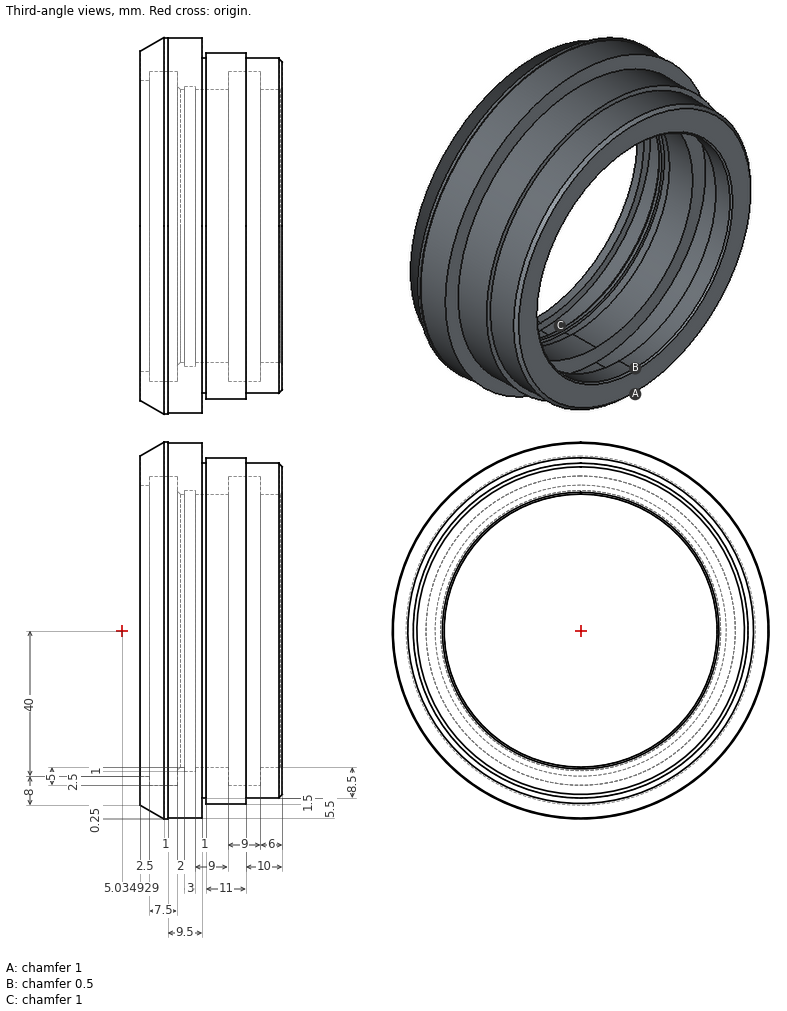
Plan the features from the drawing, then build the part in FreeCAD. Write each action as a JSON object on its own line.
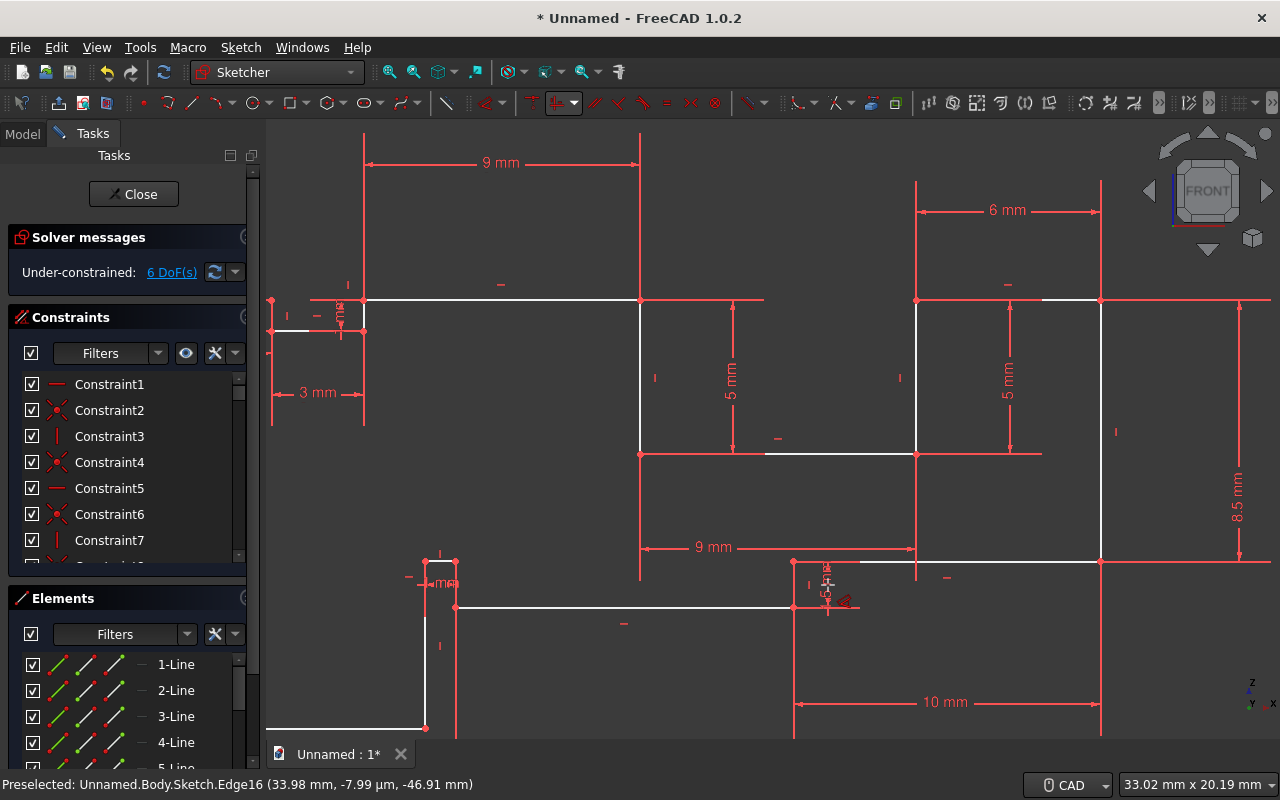
{"action": "left_click", "coordinate": [456, 594]}
{"action": "left_click", "coordinate": [514, 584]}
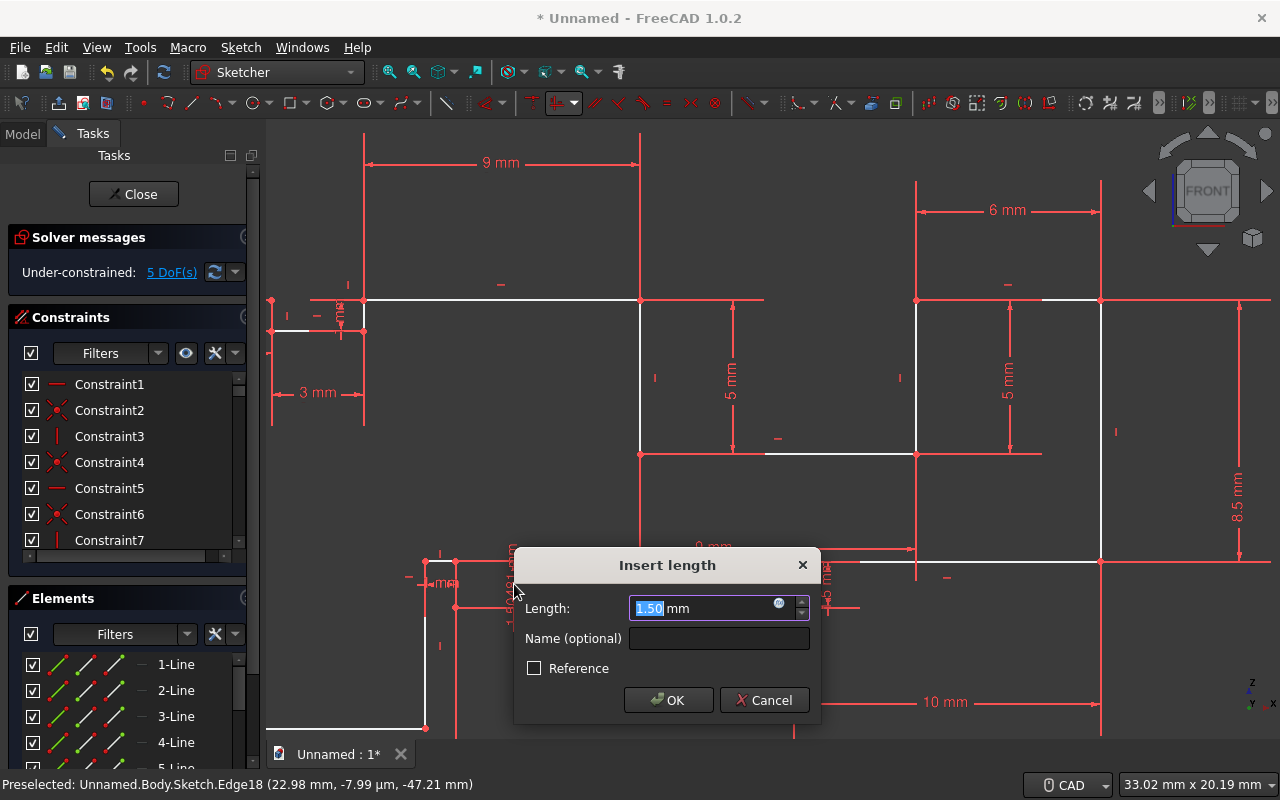
{"action": "type", "text": "1.5"}
{"action": "key", "text": "Return"}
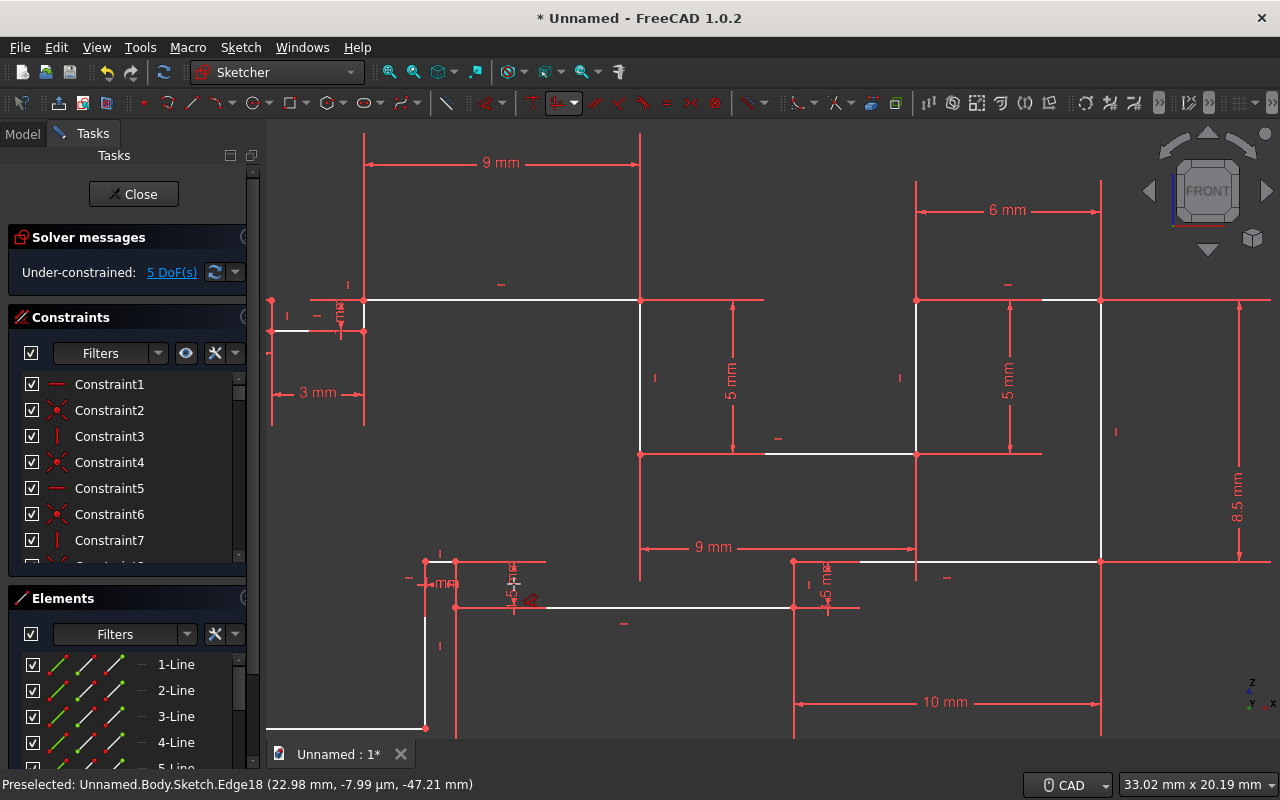
{"action": "left_click", "coordinate": [425, 612]}
{"action": "left_click", "coordinate": [391, 636]}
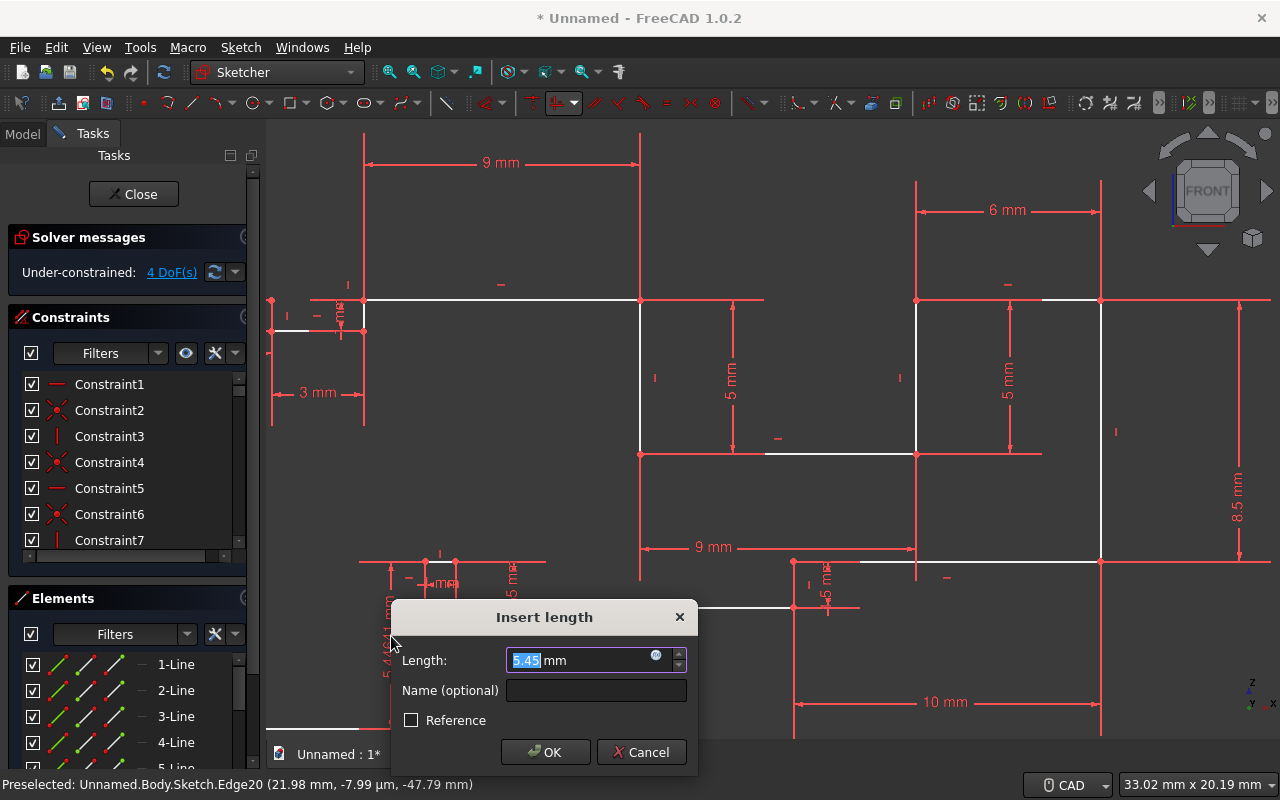
{"action": "type", "text": "5.5"}
{"action": "key", "text": "Return"}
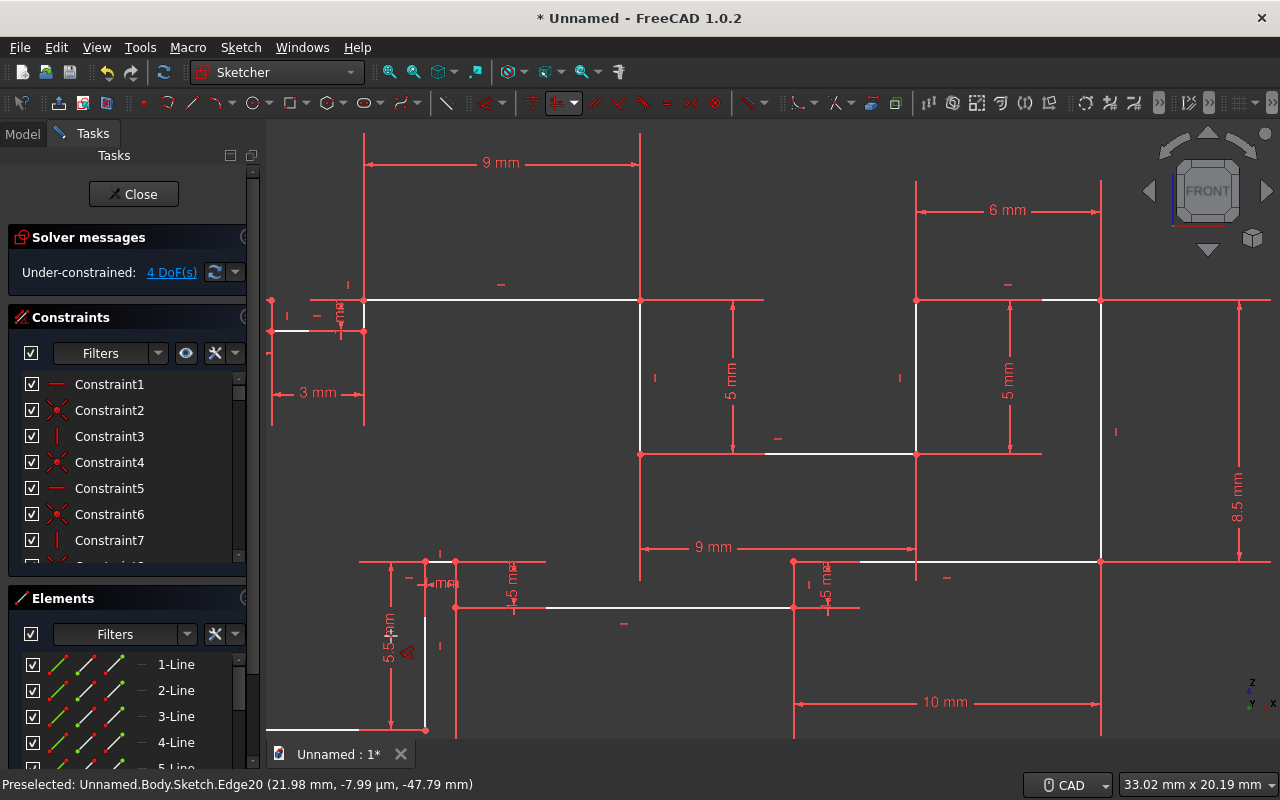
{"action": "scroll", "coordinate": [796, 589], "scroll_direction": "down", "scroll_amount": 7}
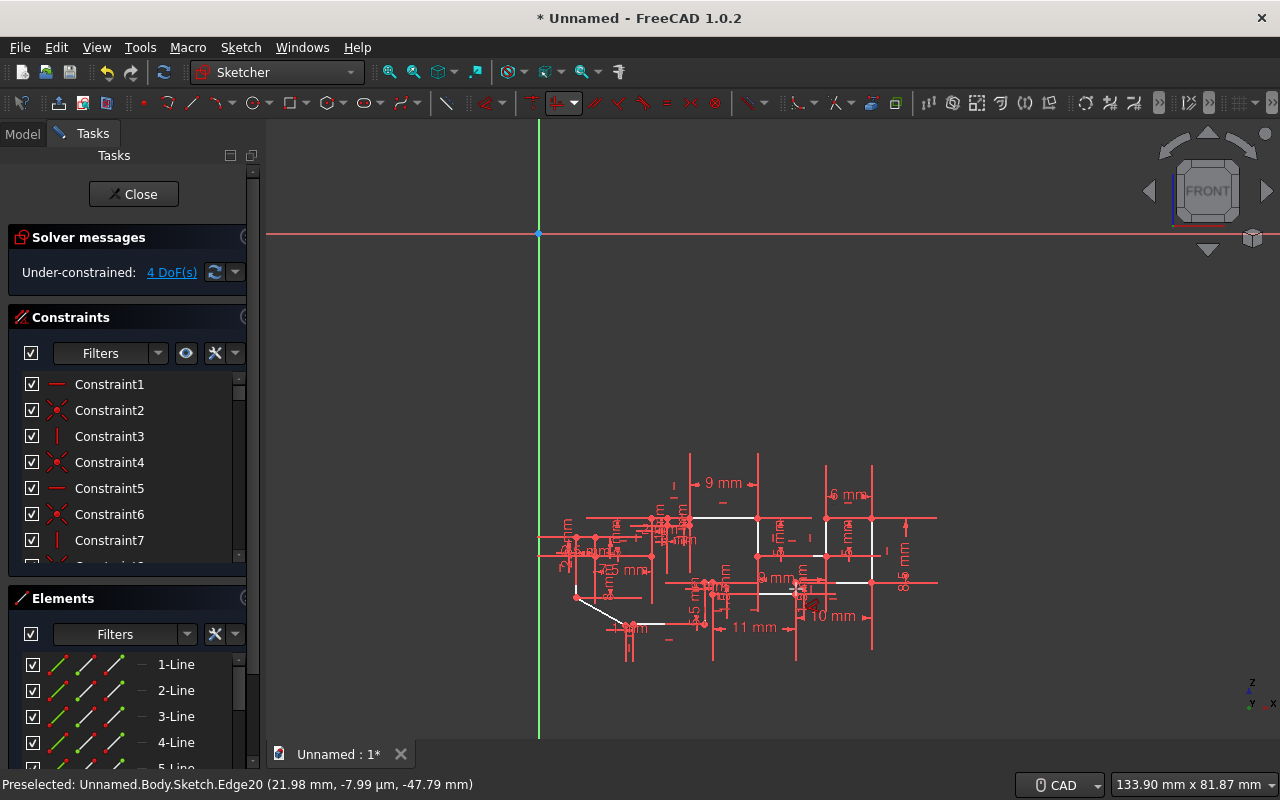
{"action": "left_click", "coordinate": [683, 624]}
{"action": "left_click", "coordinate": [669, 658]}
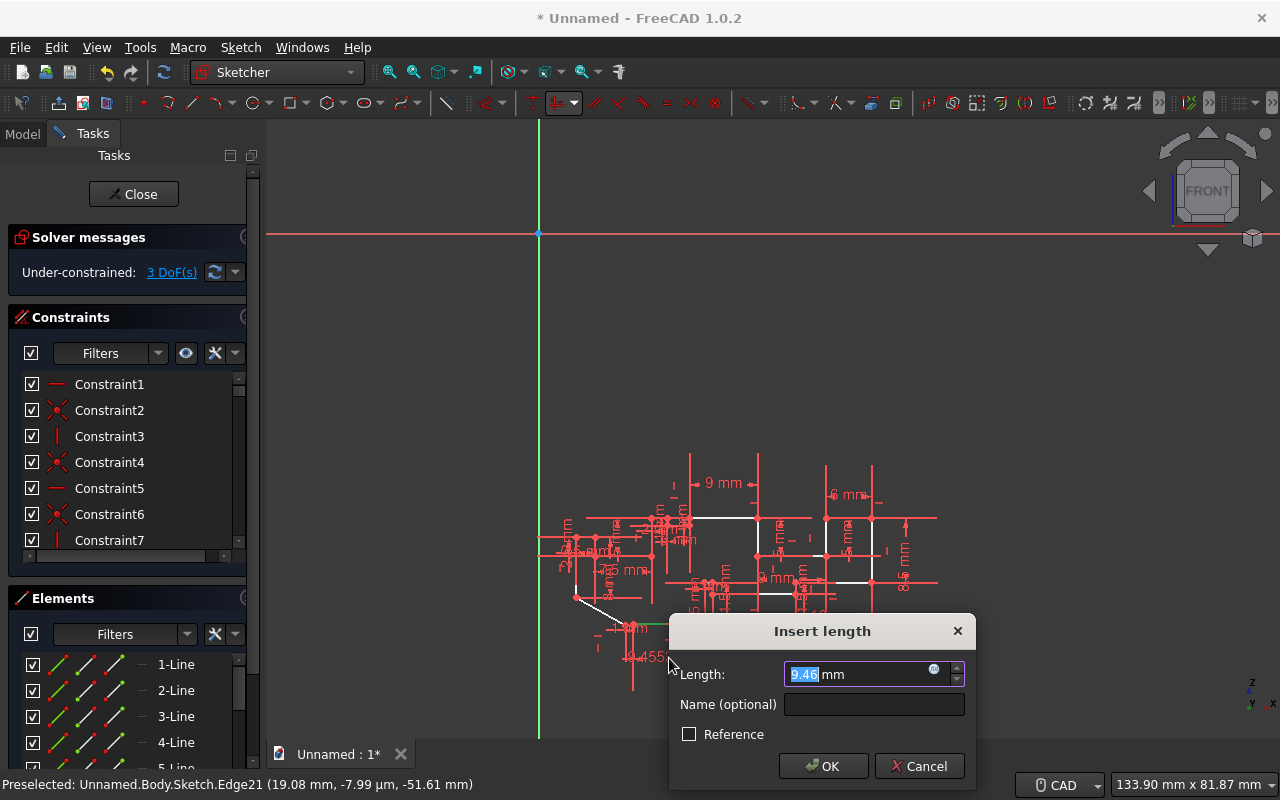
{"action": "type", "text": "9.5"}
{"action": "key", "text": "Return"}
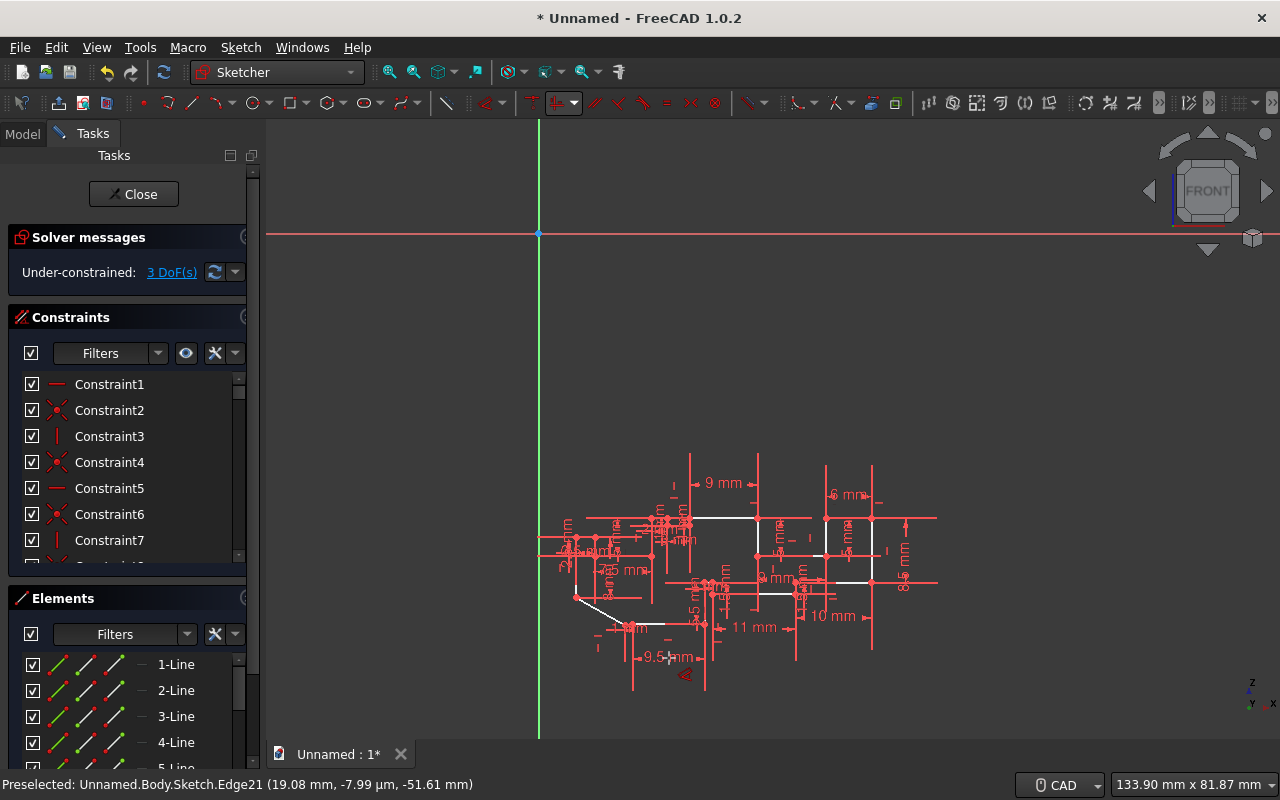
{"action": "left_click", "coordinate": [576, 537]}
{"action": "left_click", "coordinate": [505, 385]}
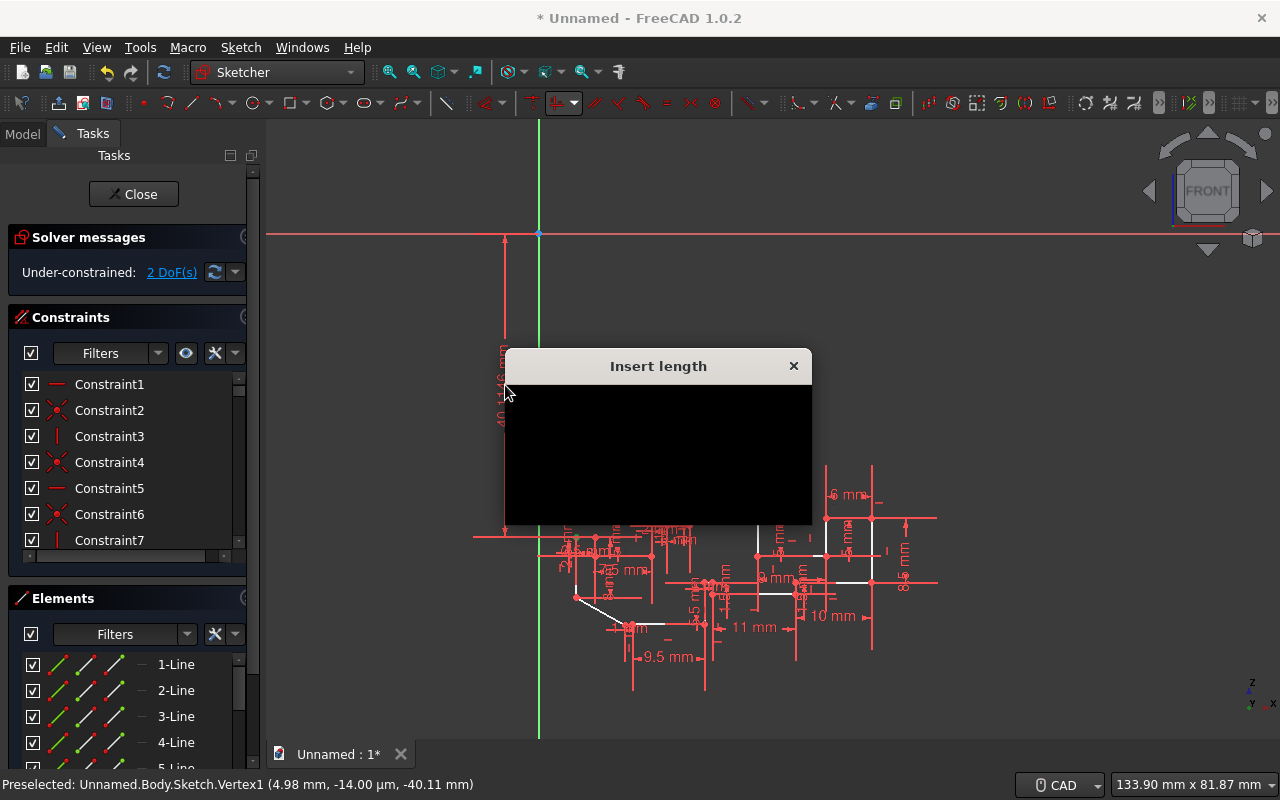
{"action": "type", "text": "40"}
{"action": "key", "text": "Return"}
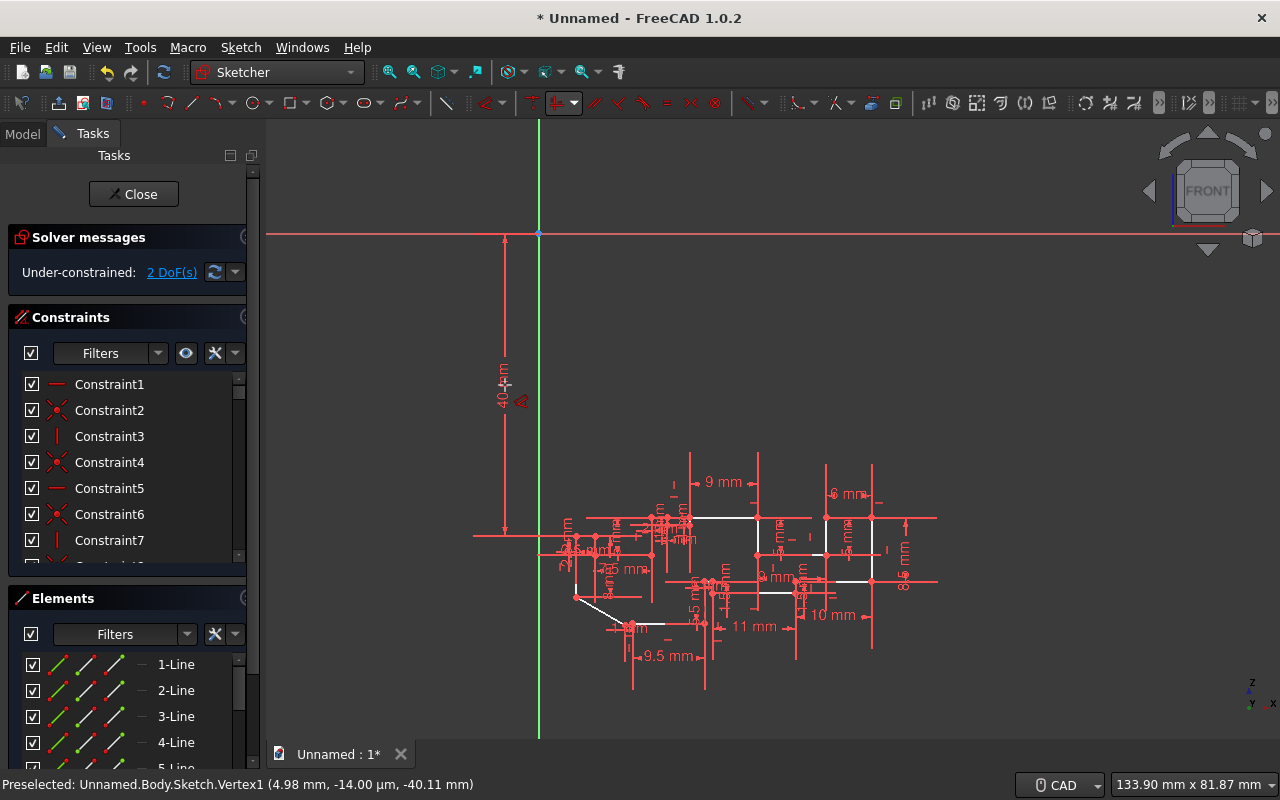
{"action": "scroll", "coordinate": [633, 625], "scroll_direction": "up", "scroll_amount": 16}